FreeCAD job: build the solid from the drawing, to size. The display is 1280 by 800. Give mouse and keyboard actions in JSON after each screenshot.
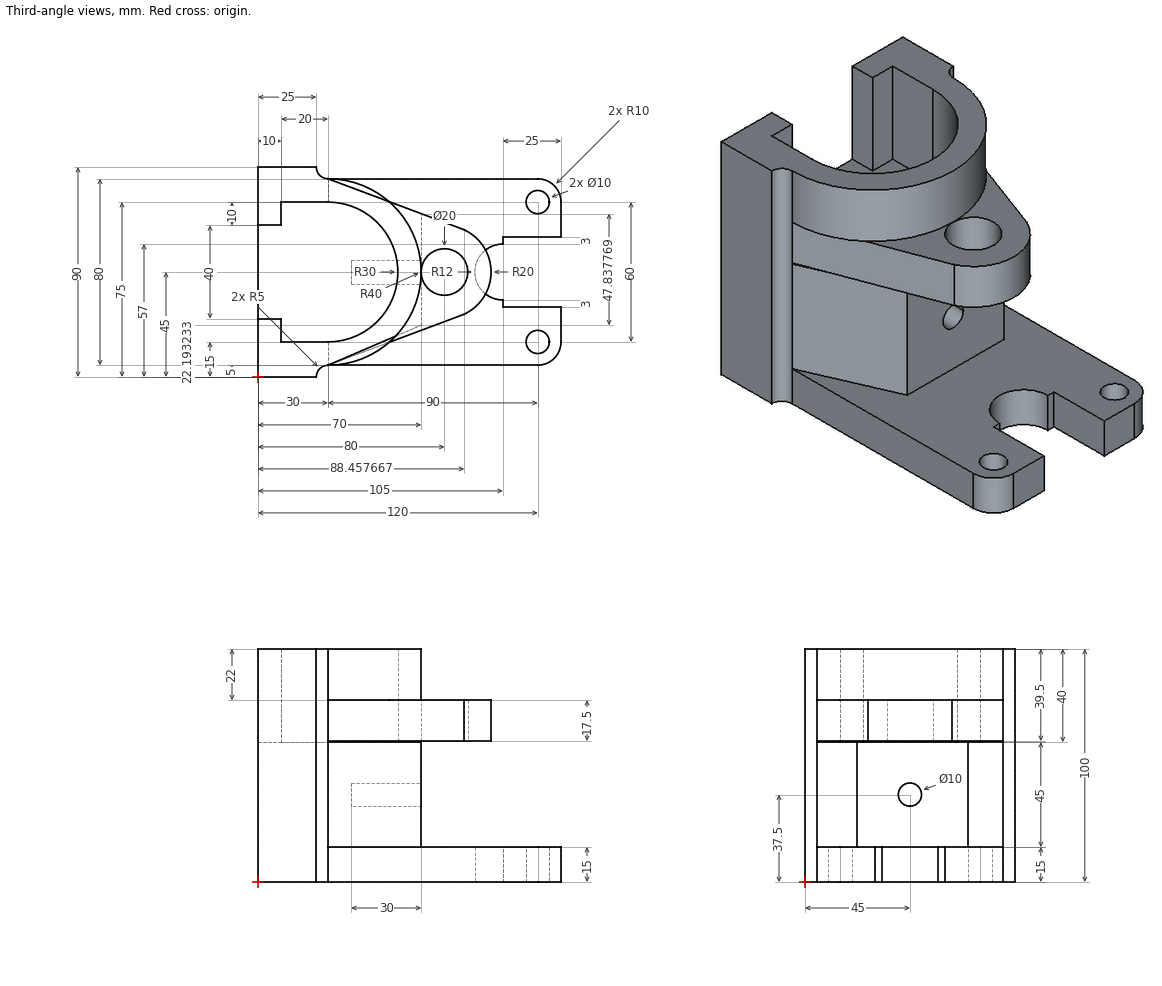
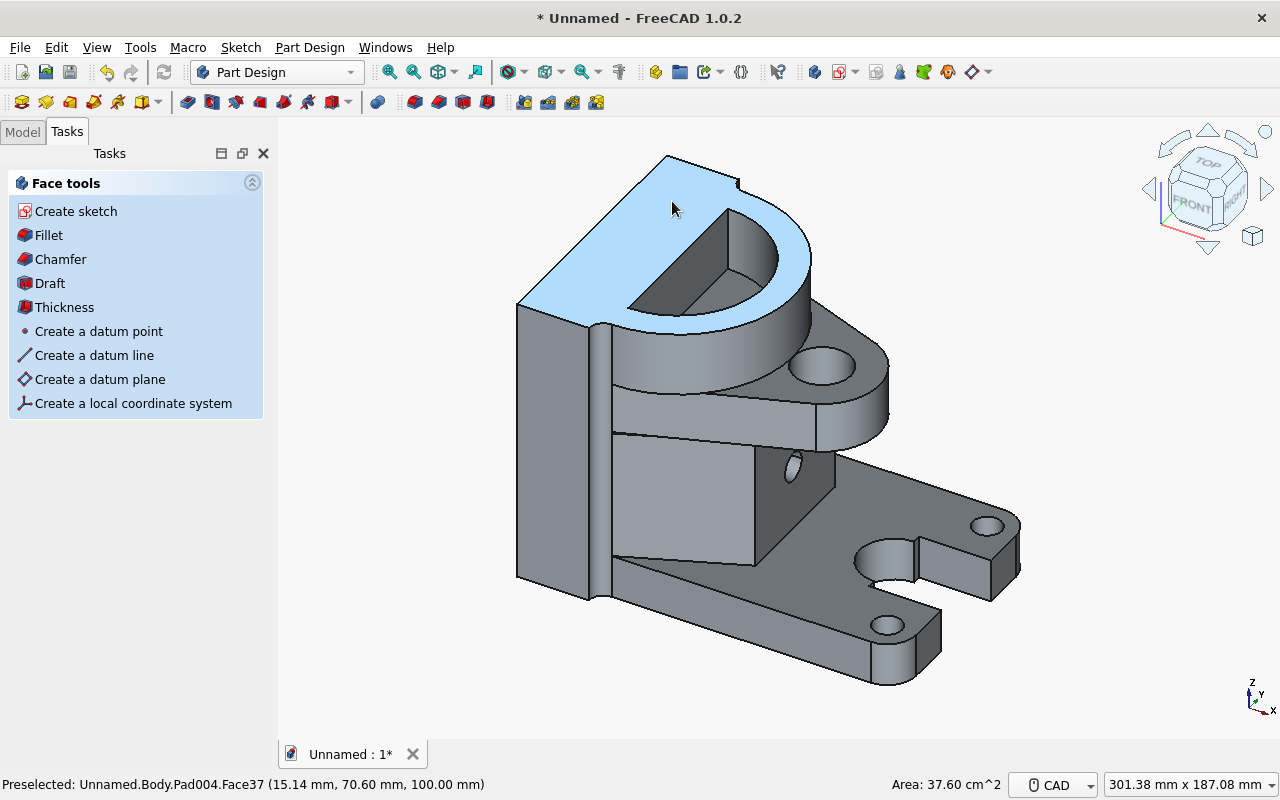
{"action": "left_click", "coordinate": [840, 72]}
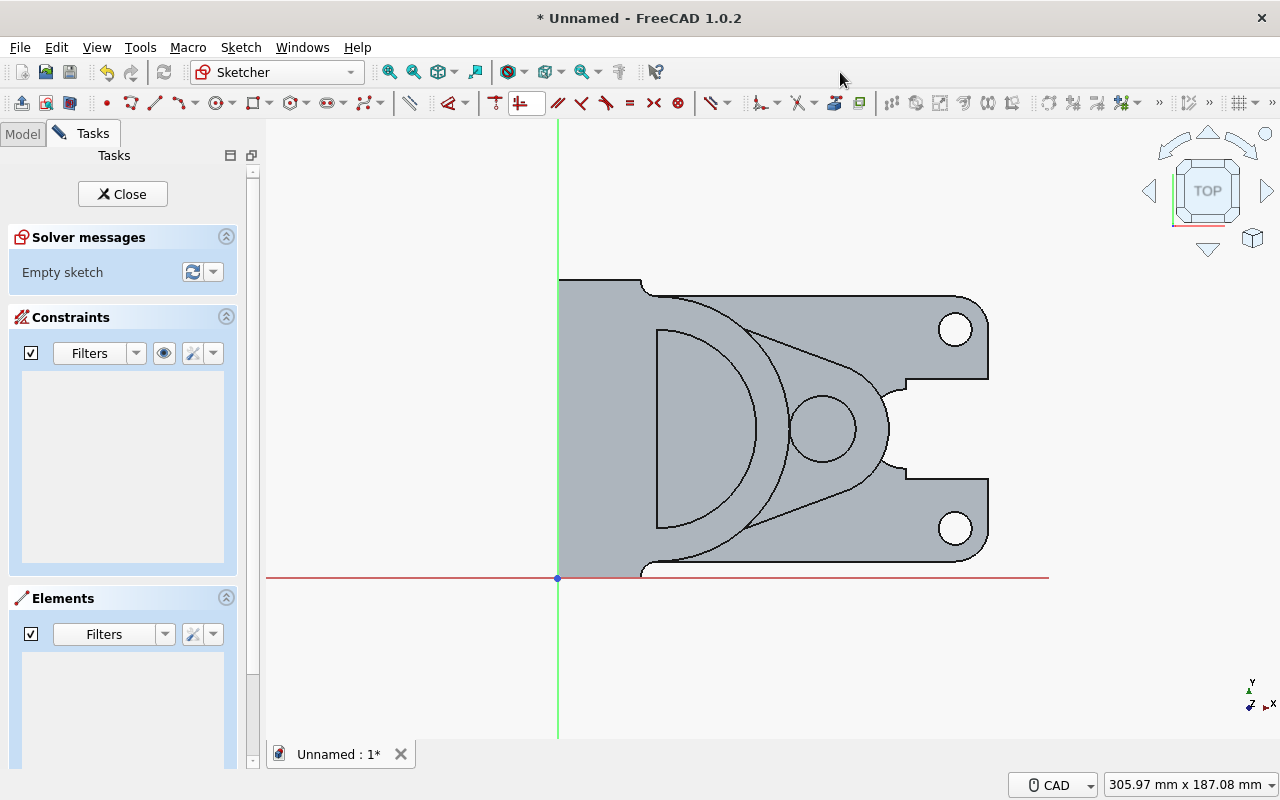
{"action": "scroll", "coordinate": [560, 504], "scroll_direction": "up", "scroll_amount": 2}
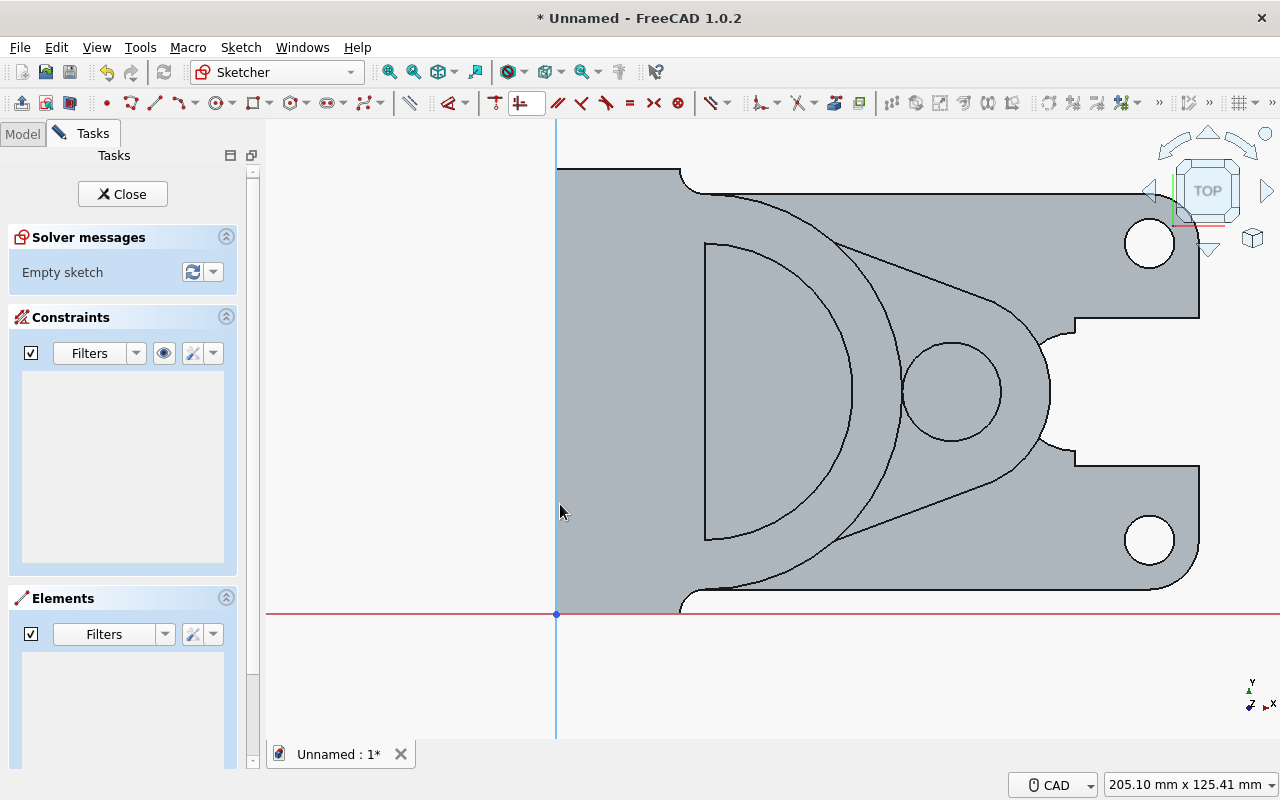
{"action": "left_click", "coordinate": [132, 104]}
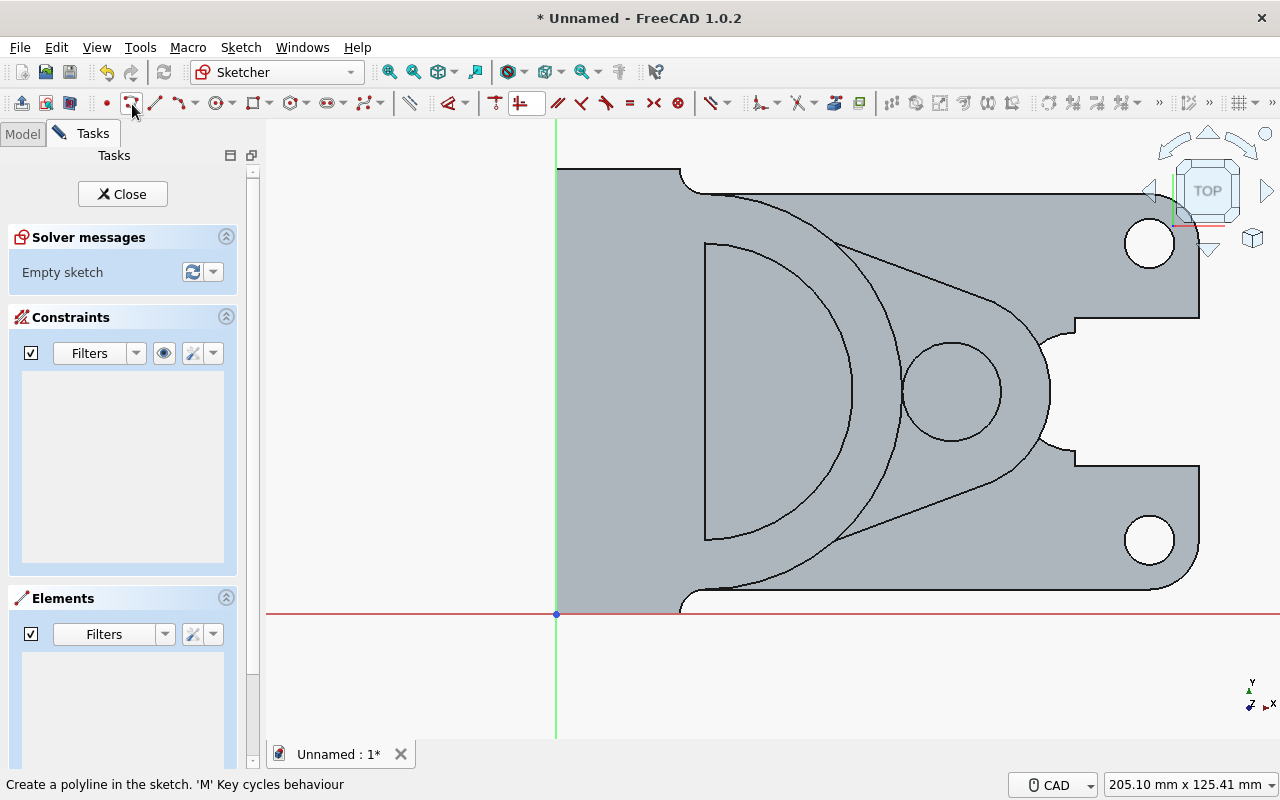
{"action": "left_click", "coordinate": [705, 243]}
{"action": "left_click", "coordinate": [606, 243]}
{"action": "left_click", "coordinate": [606, 293]}
{"action": "left_click", "coordinate": [556, 293]}
{"action": "left_click", "coordinate": [565, 491]}
{"action": "left_click", "coordinate": [606, 491]}
{"action": "left_click", "coordinate": [606, 540]}
{"action": "left_click", "coordinate": [705, 540]}
{"action": "right_click", "coordinate": [705, 540]}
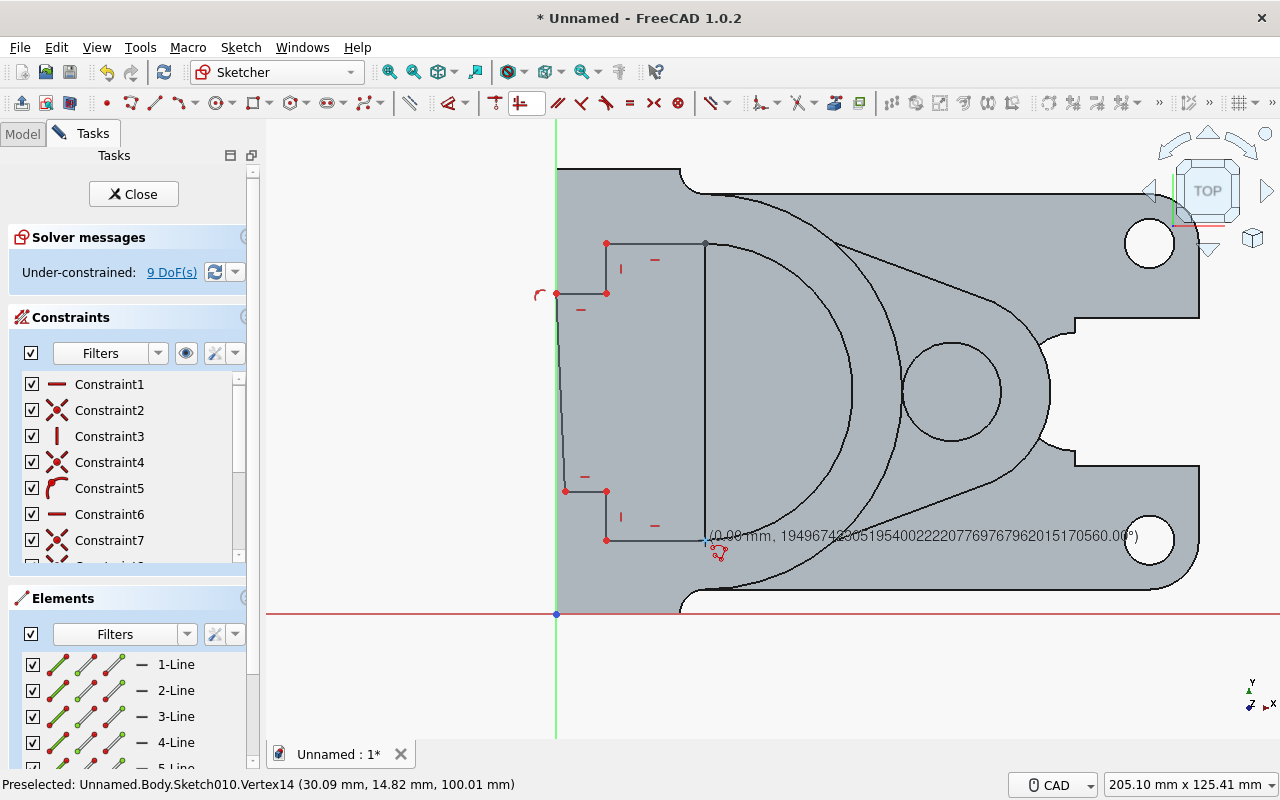
{"action": "left_click", "coordinate": [180, 104]}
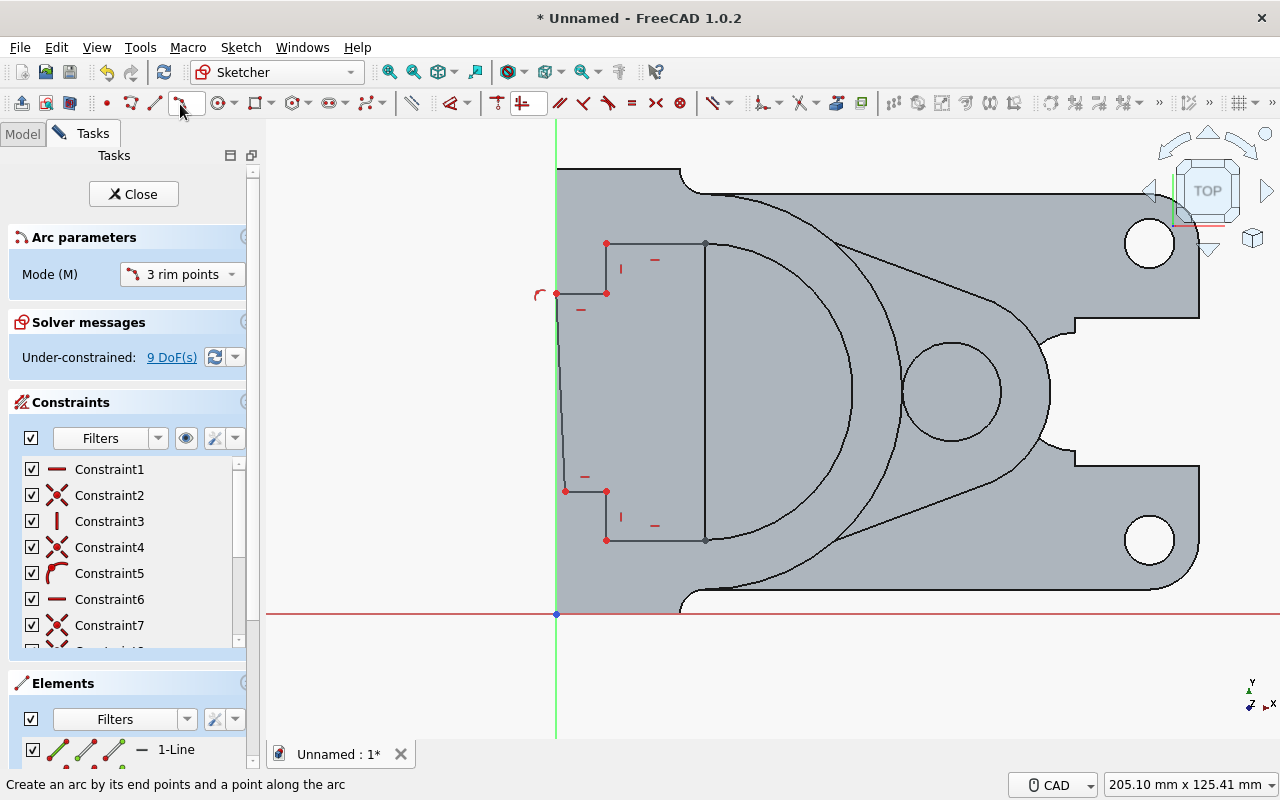
{"action": "left_click", "coordinate": [705, 541]}
{"action": "left_click", "coordinate": [705, 244]}
{"action": "left_click", "coordinate": [853, 392]}
{"action": "key", "text": "Escape"}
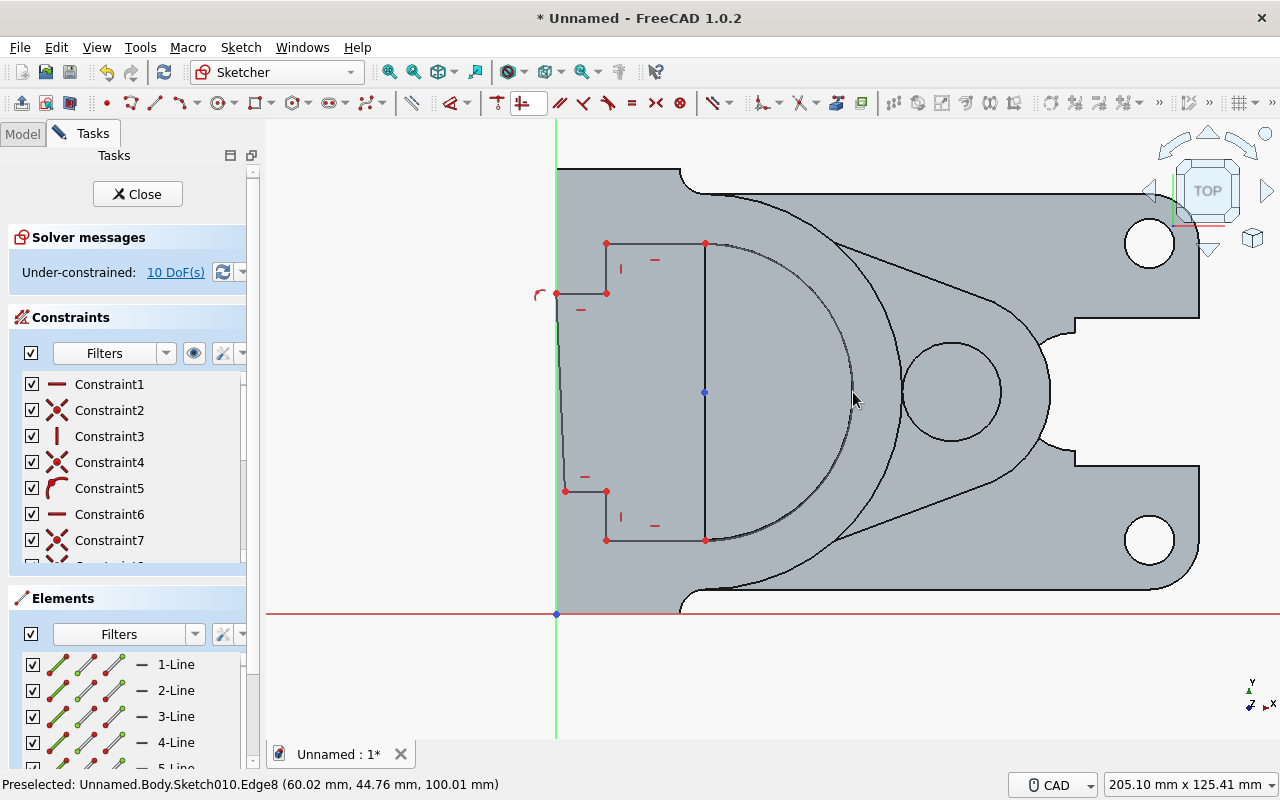
{"action": "left_click", "coordinate": [675, 244]}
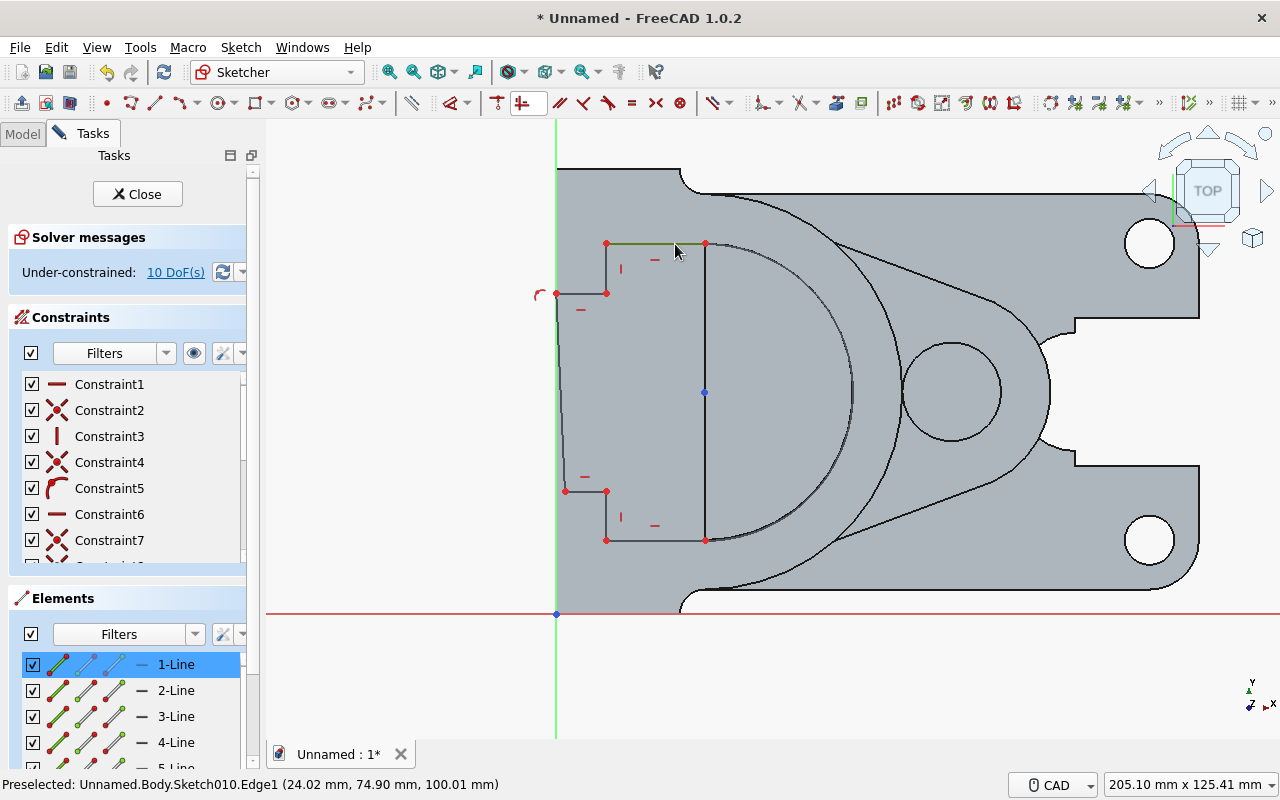
{"action": "left_click", "coordinate": [825, 480]}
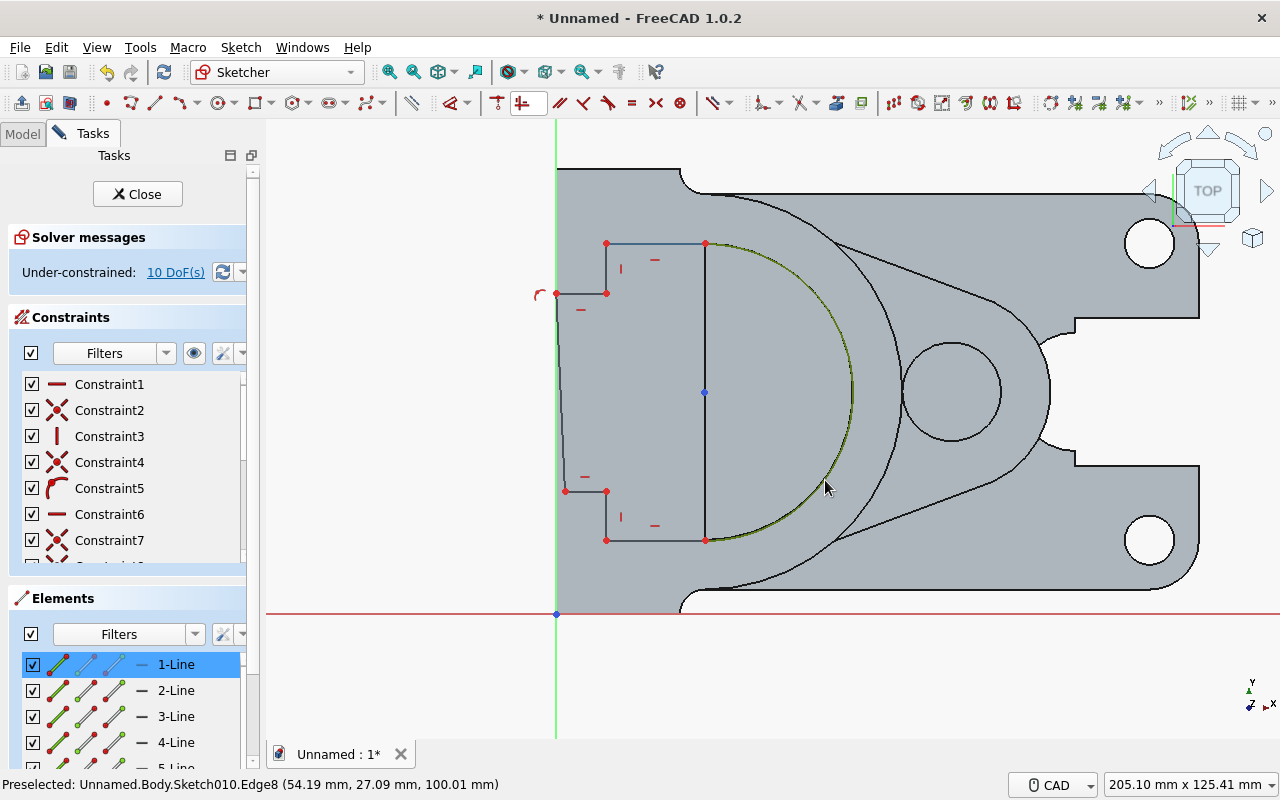
{"action": "left_click", "coordinate": [608, 104]}